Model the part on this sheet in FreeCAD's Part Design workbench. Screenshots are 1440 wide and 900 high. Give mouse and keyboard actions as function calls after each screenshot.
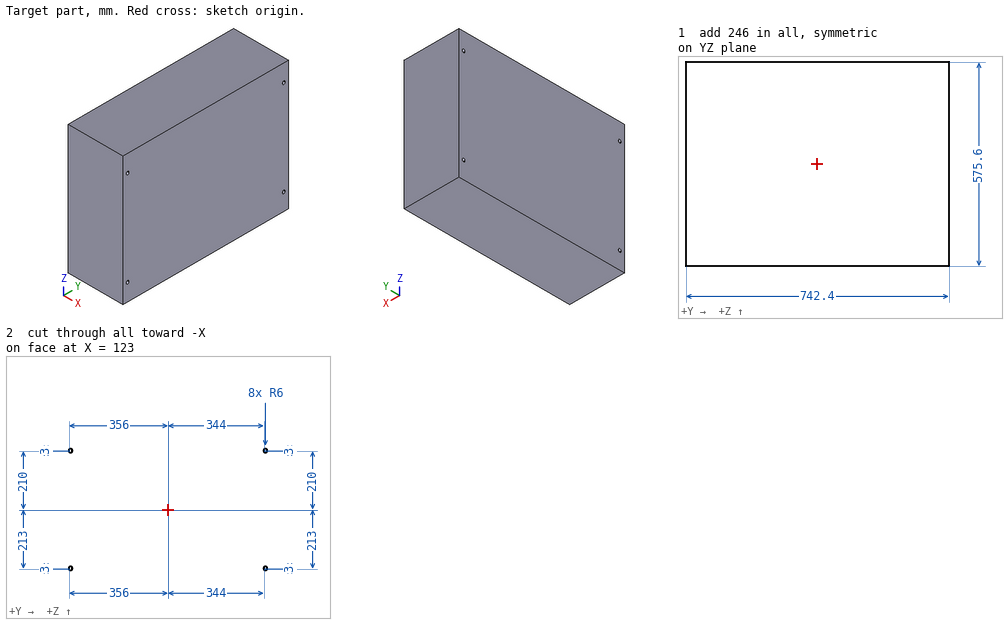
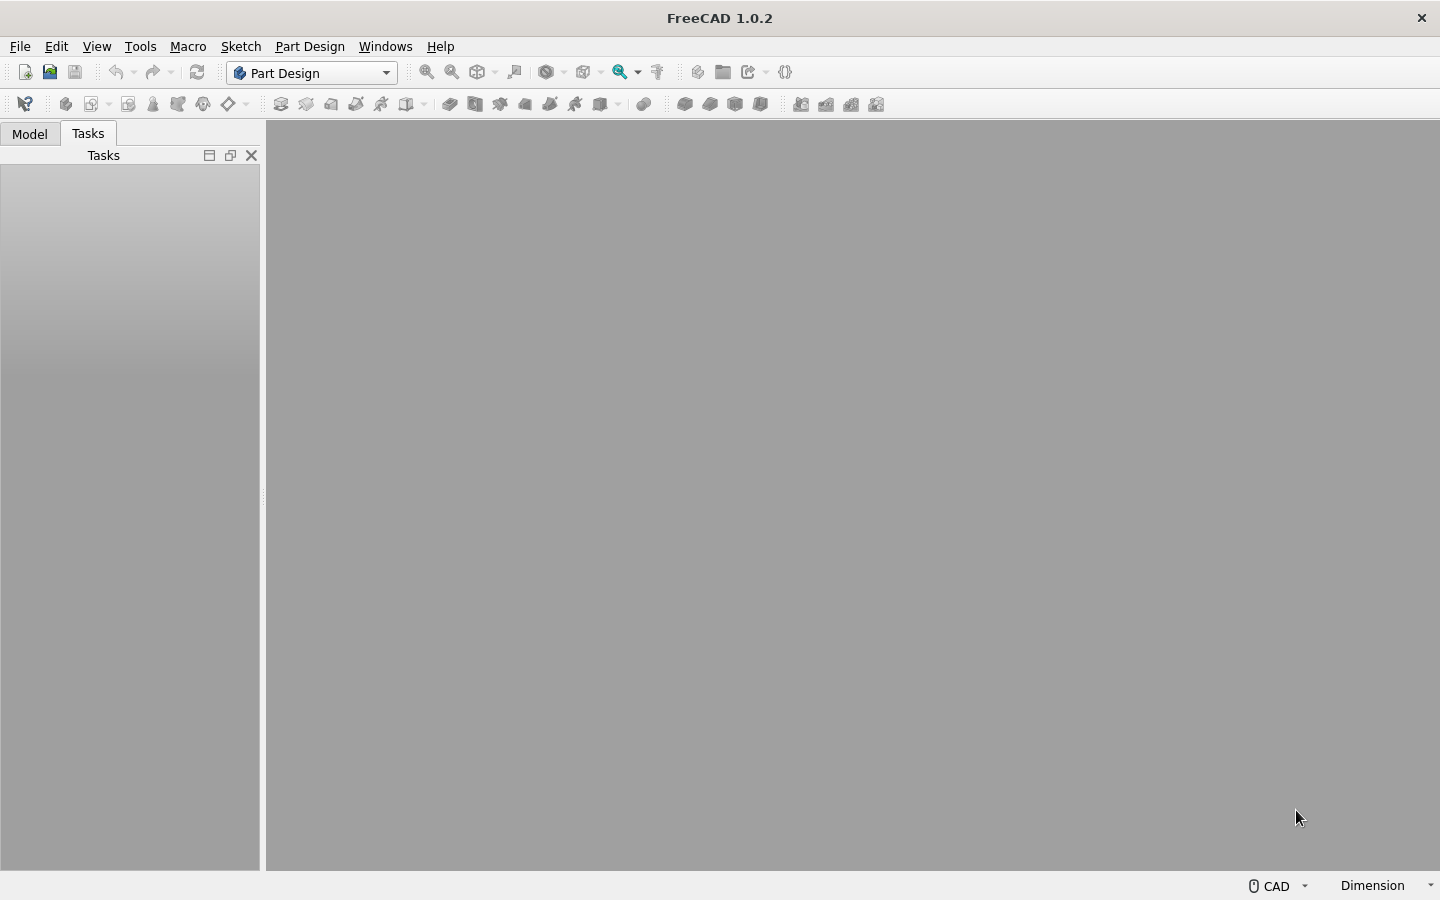
key(ctrl+n)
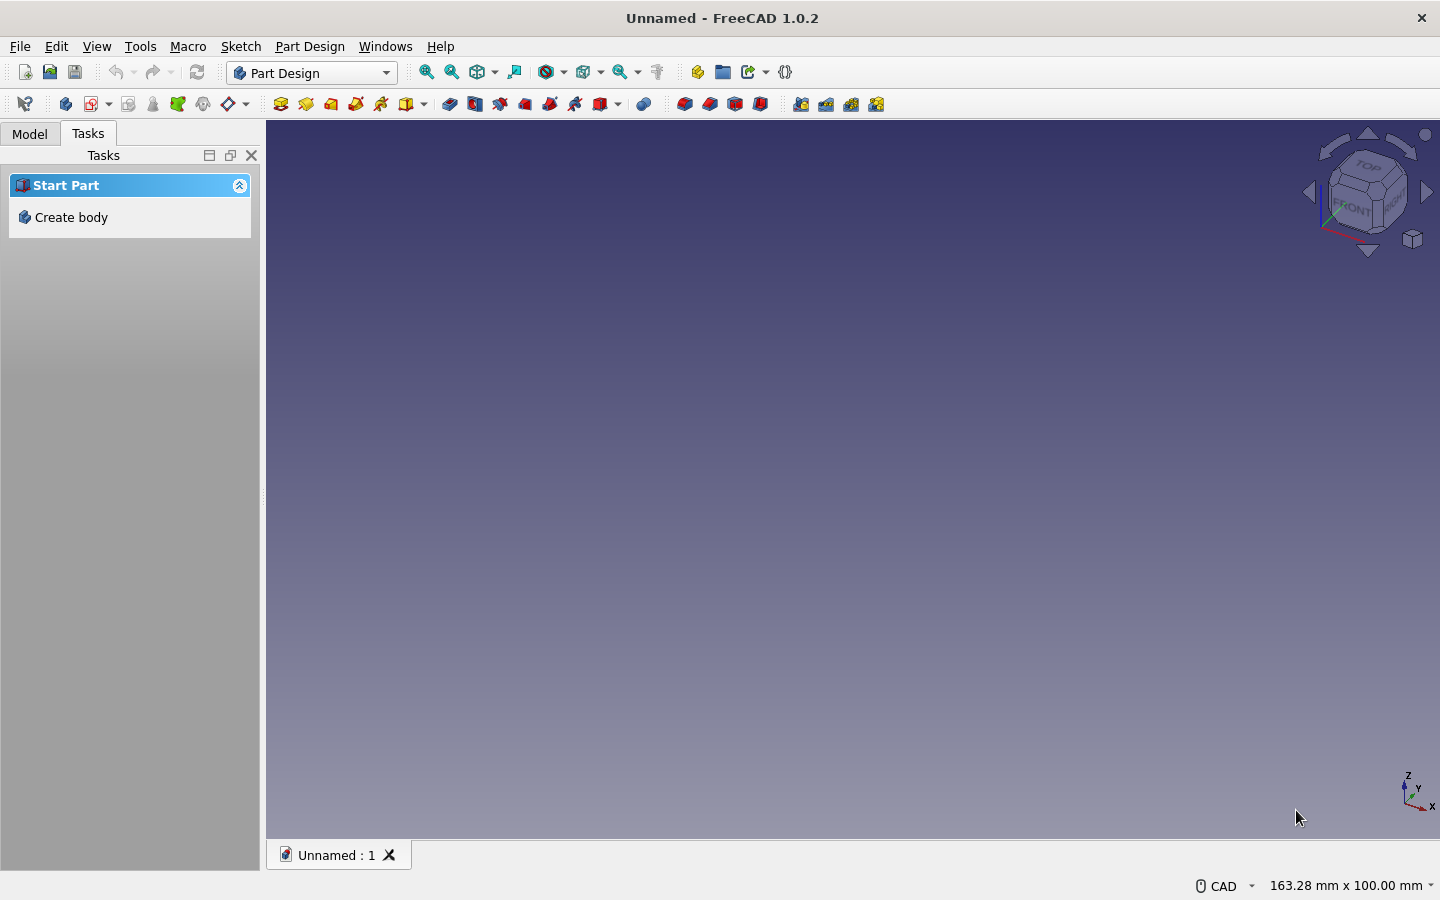
click(90, 104)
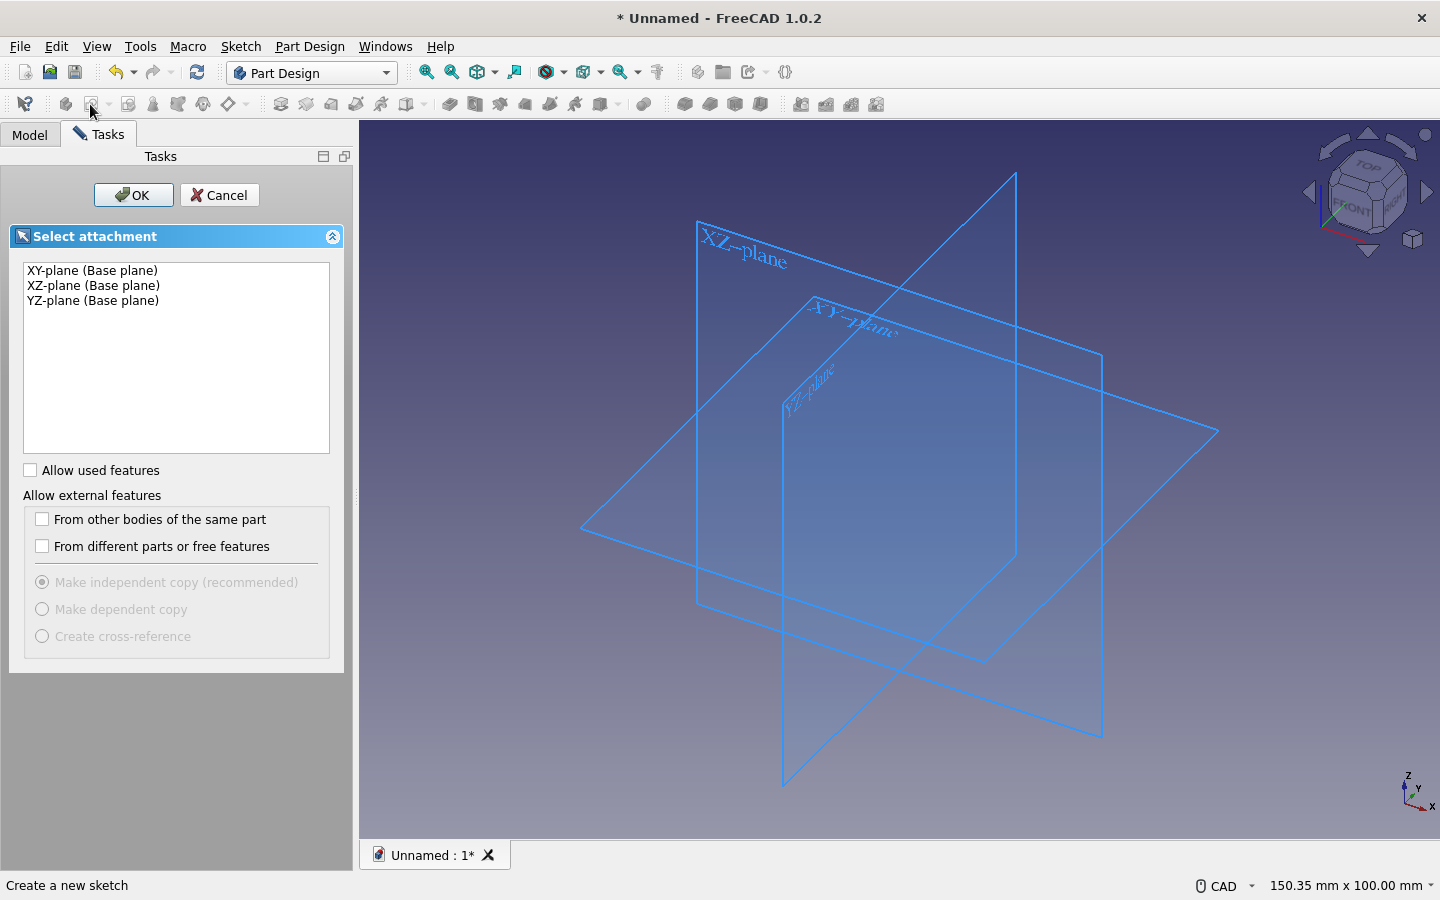
click(84, 300)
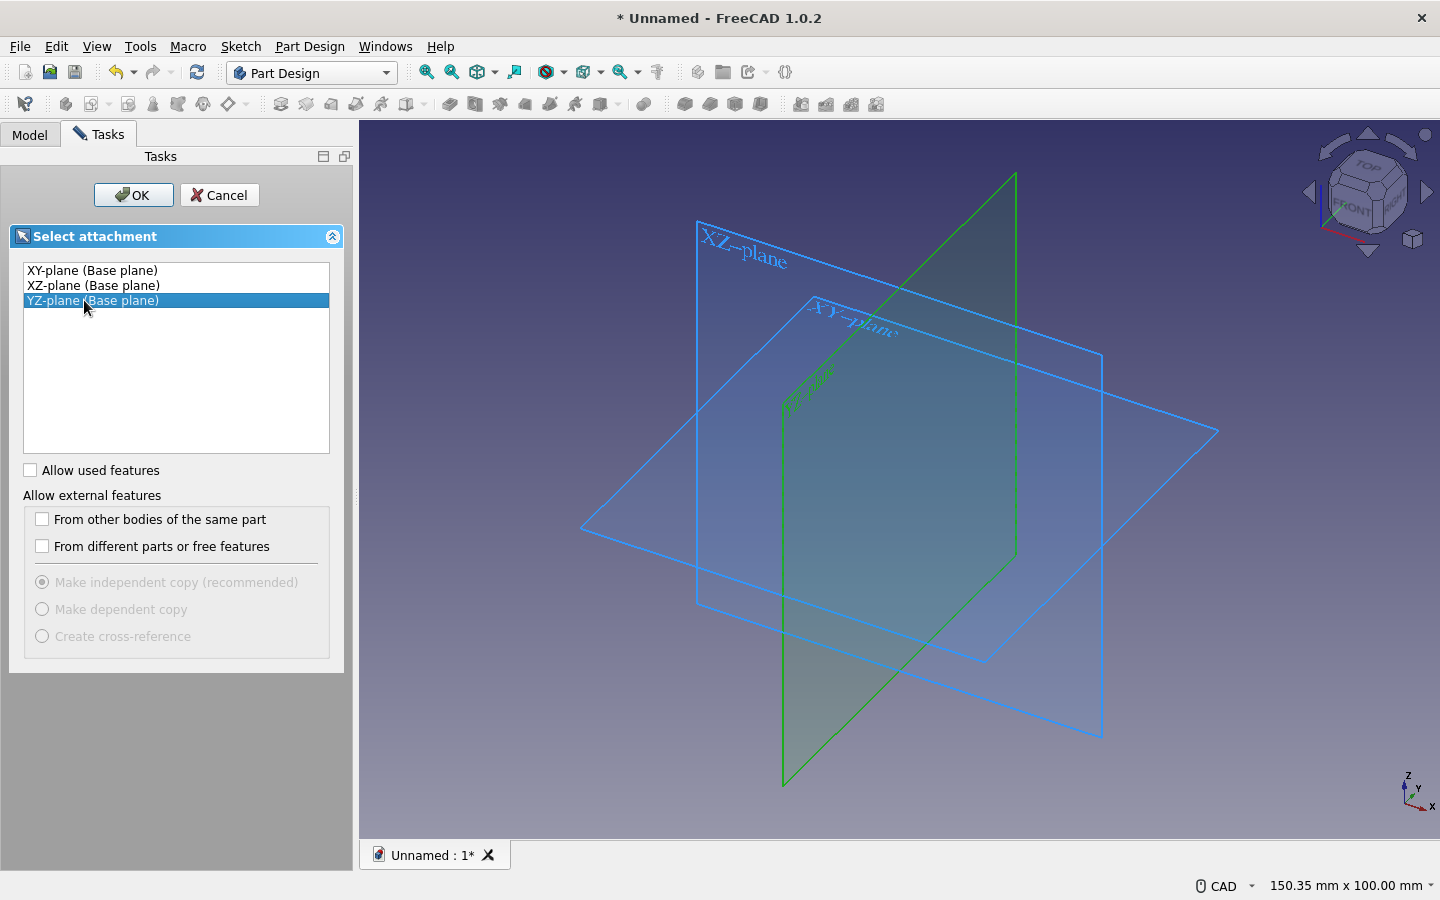
click(134, 195)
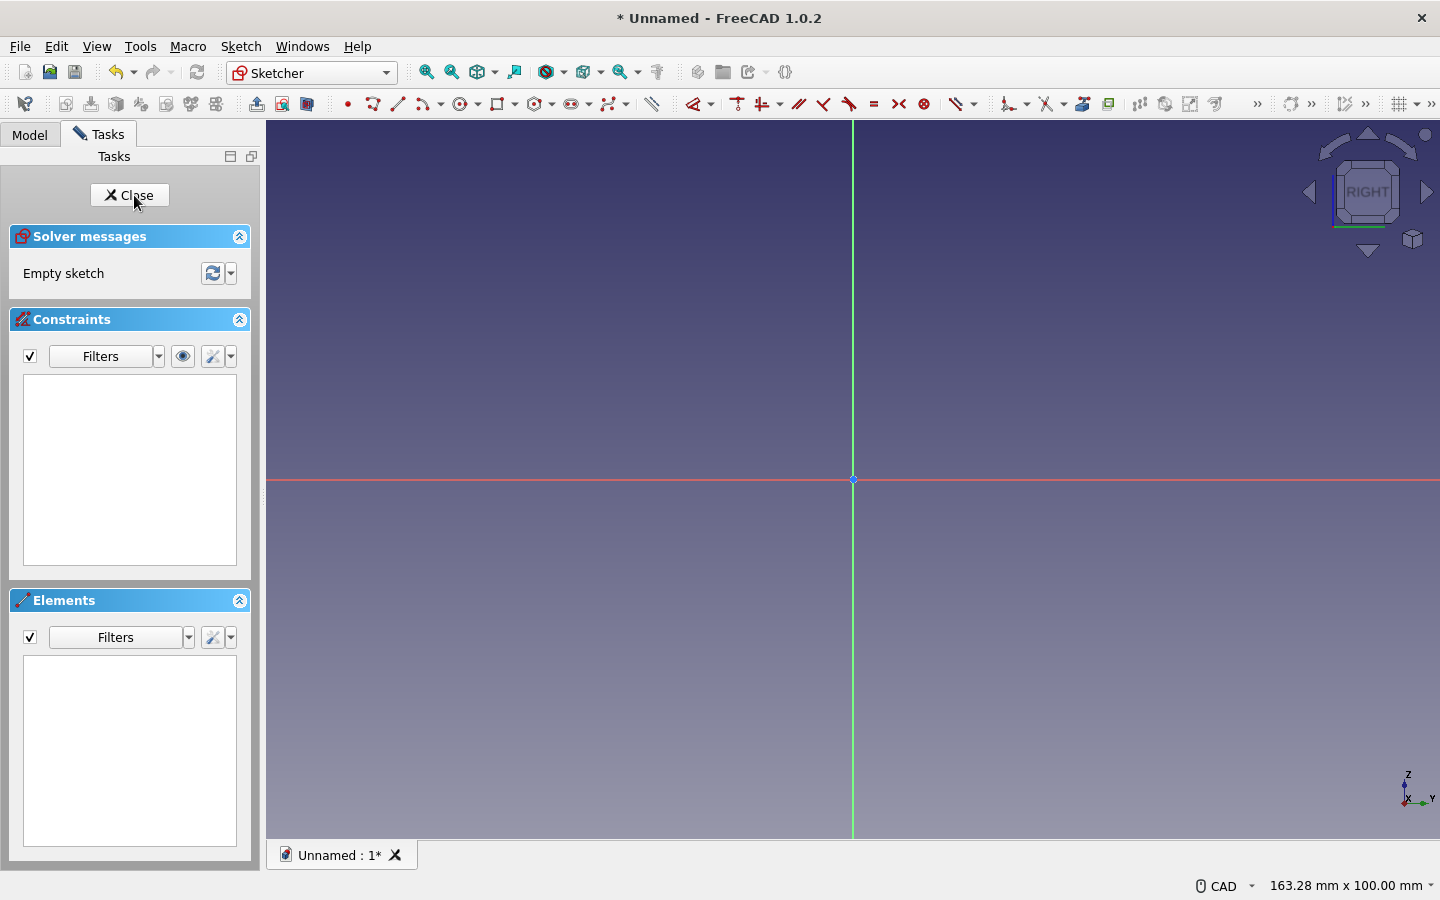
scroll(776, 480, down, 11)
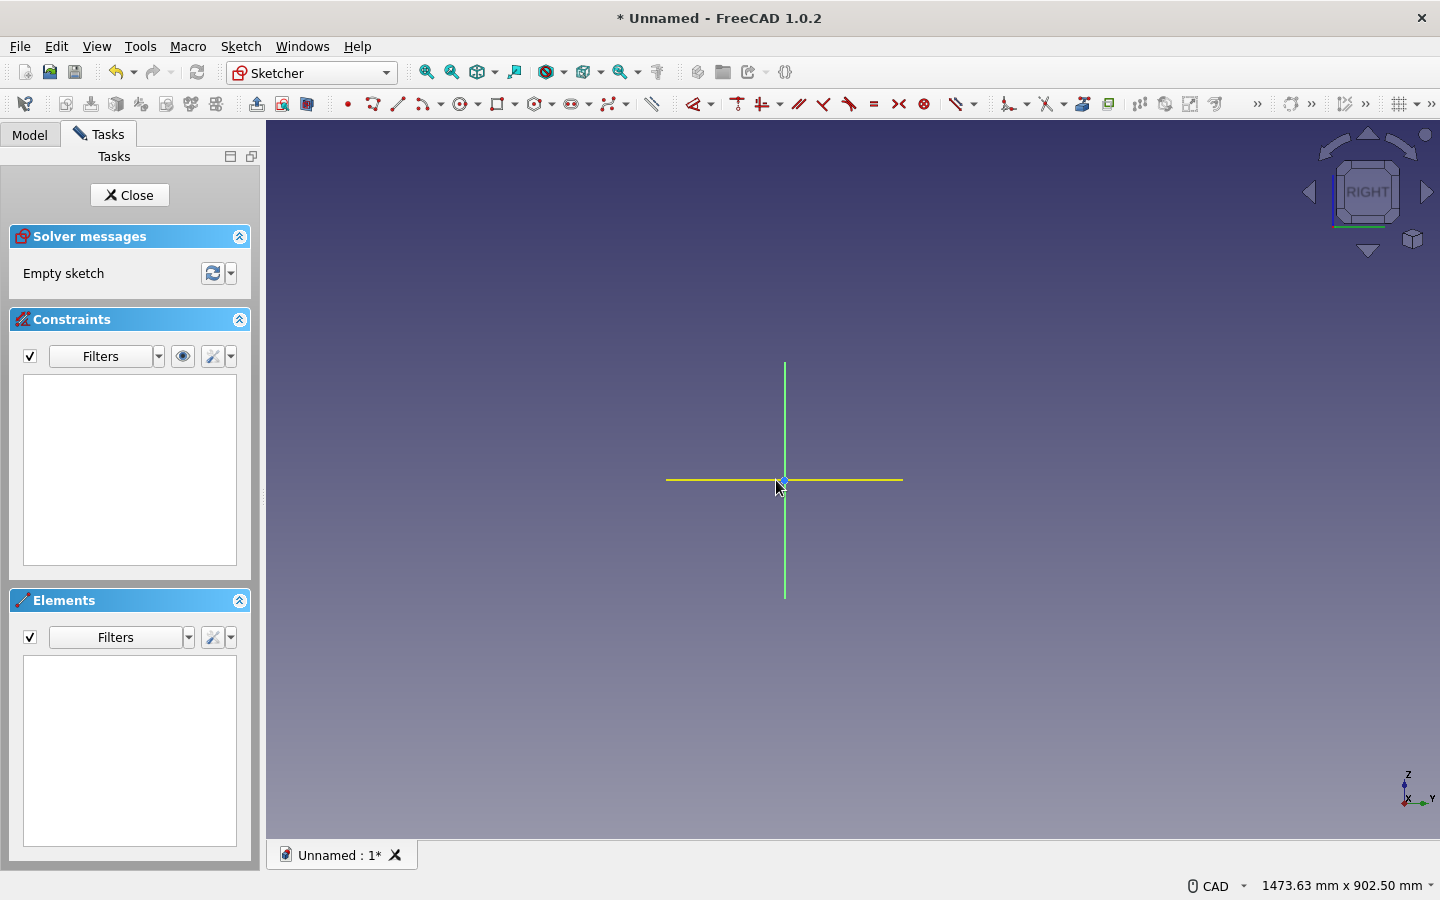
click(514, 104)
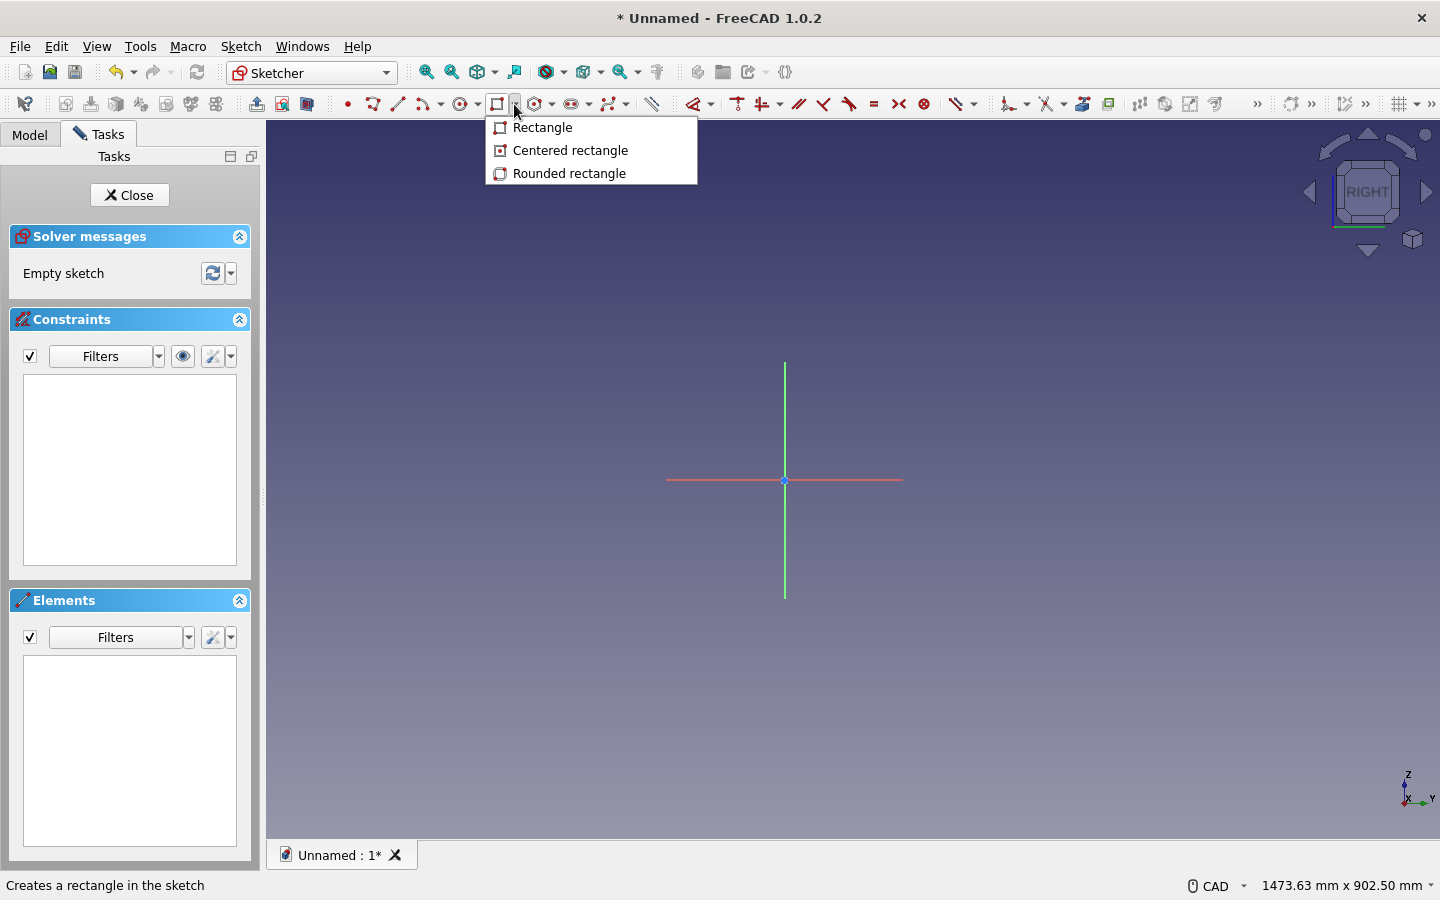
click(592, 150)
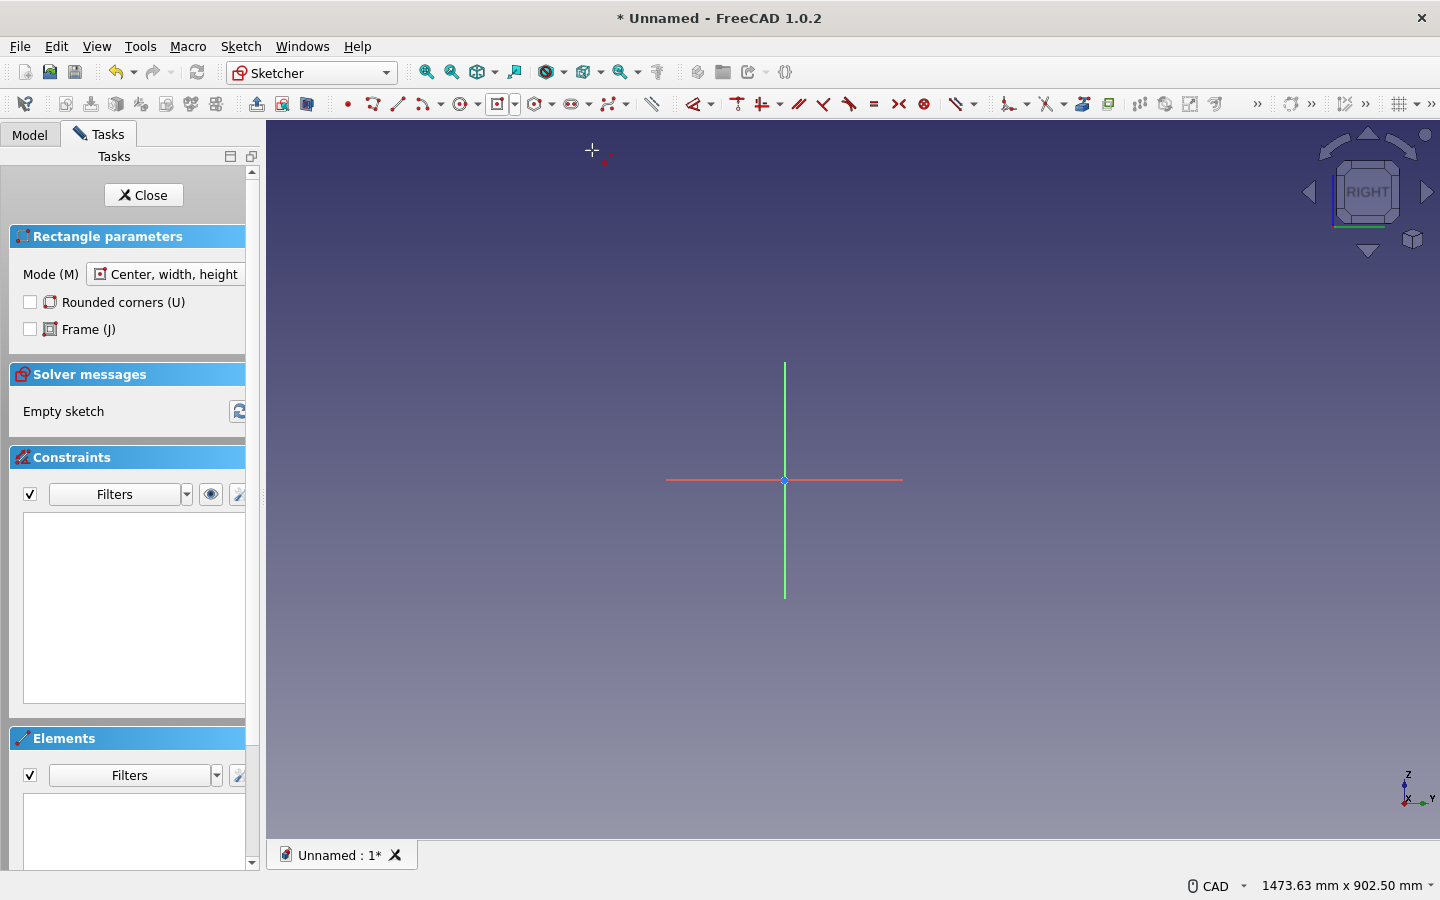
click(785, 480)
move(1081, 251)